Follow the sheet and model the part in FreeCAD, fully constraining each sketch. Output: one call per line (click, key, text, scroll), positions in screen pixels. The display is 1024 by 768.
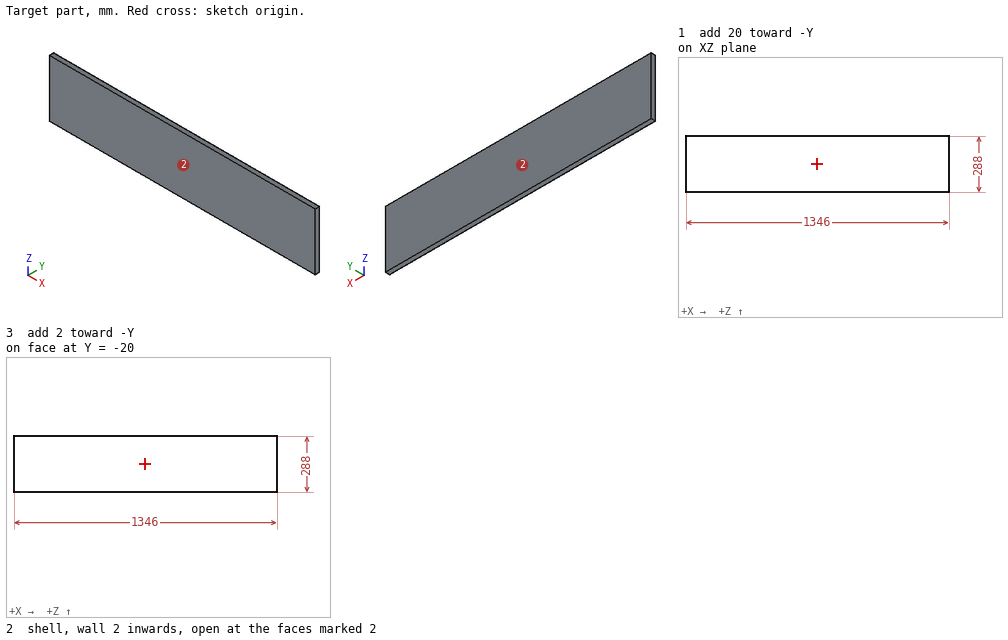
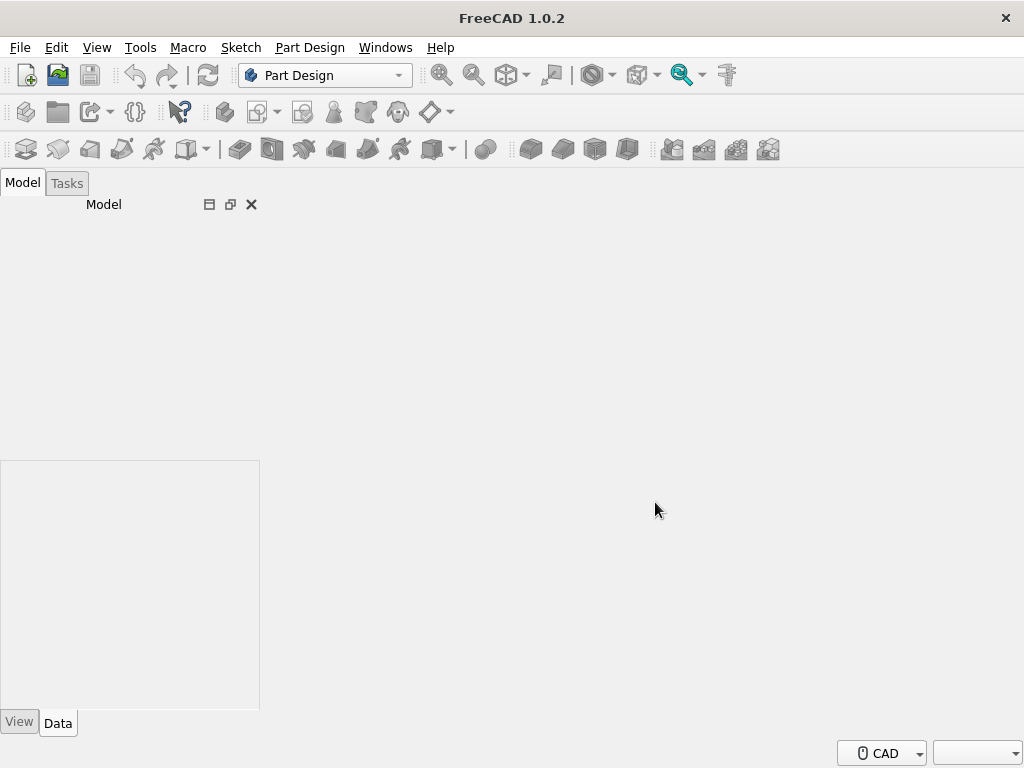
click(26, 76)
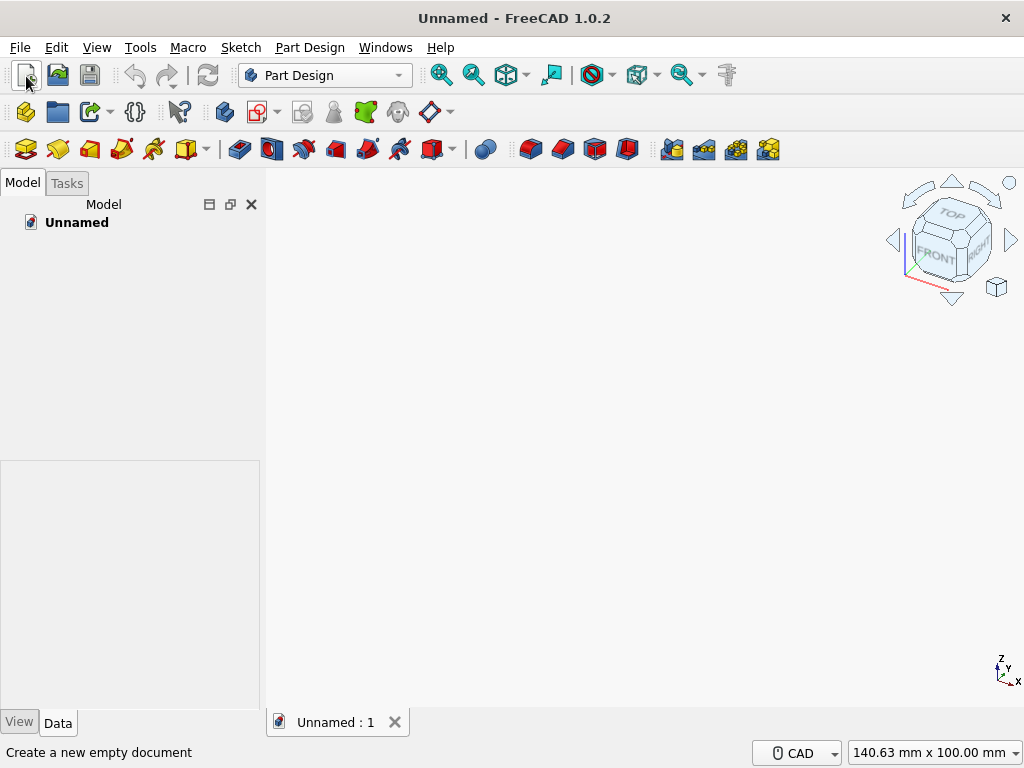
click(258, 112)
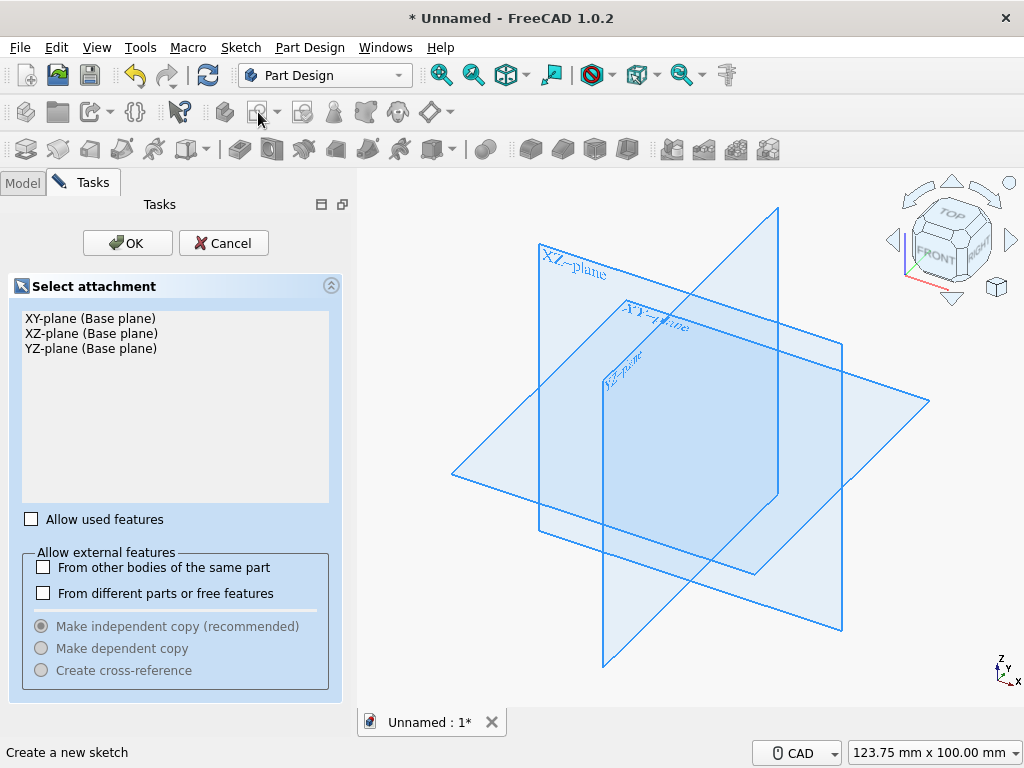
click(82, 334)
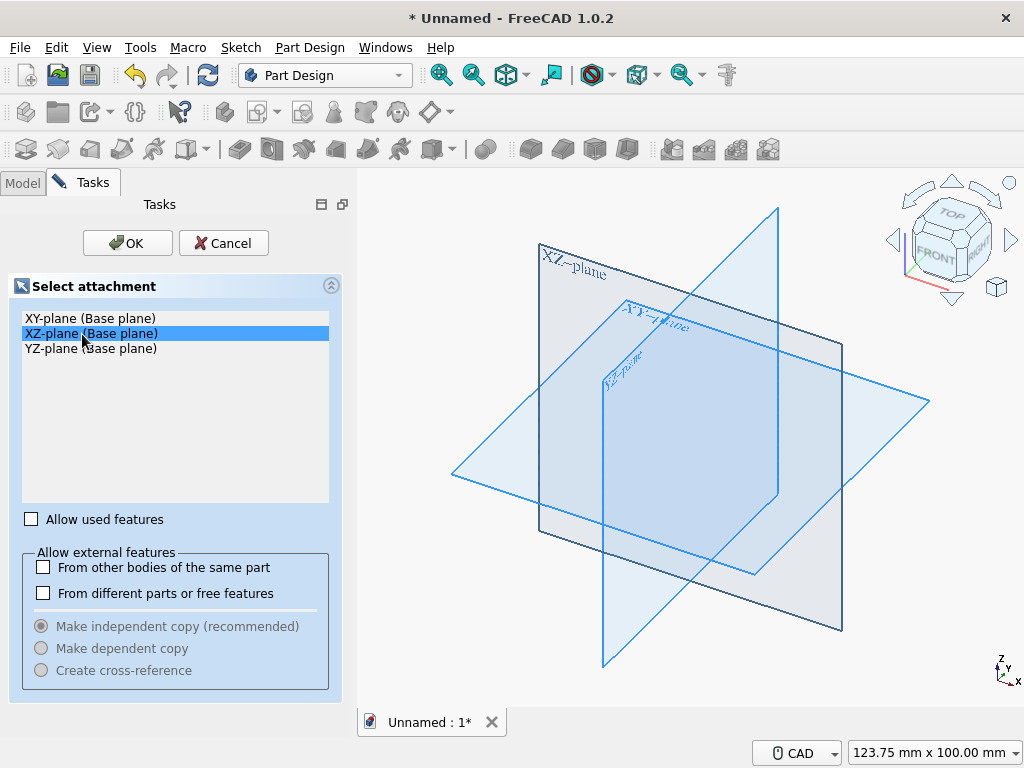
click(128, 243)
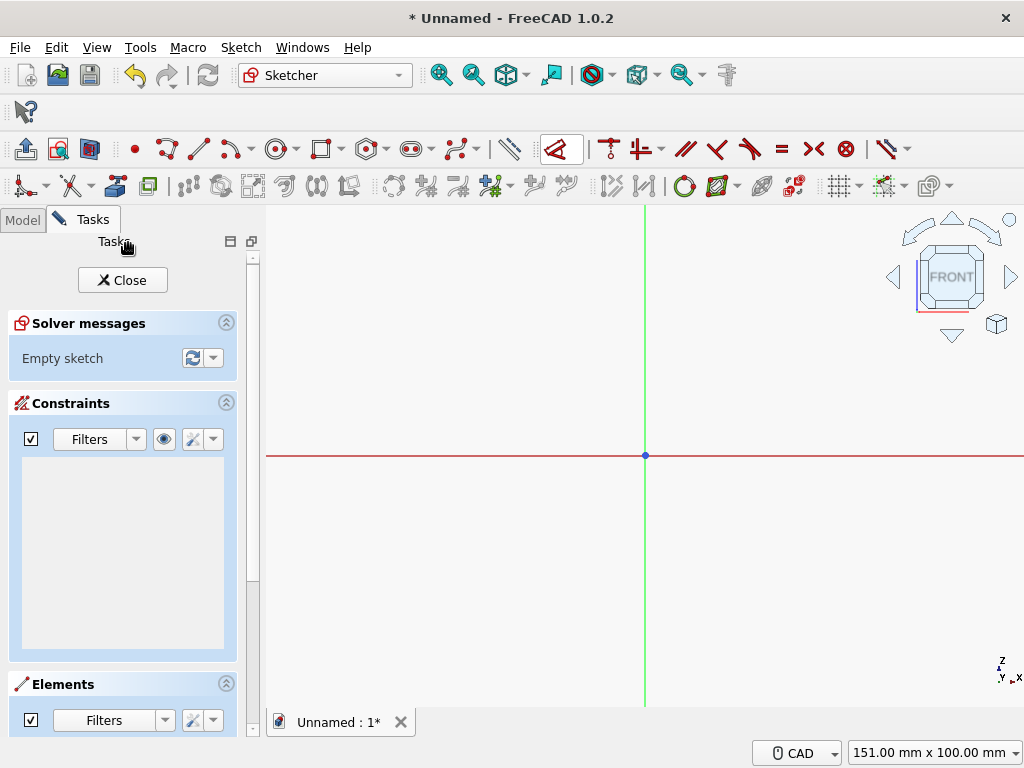
scroll(572, 456, down, 14)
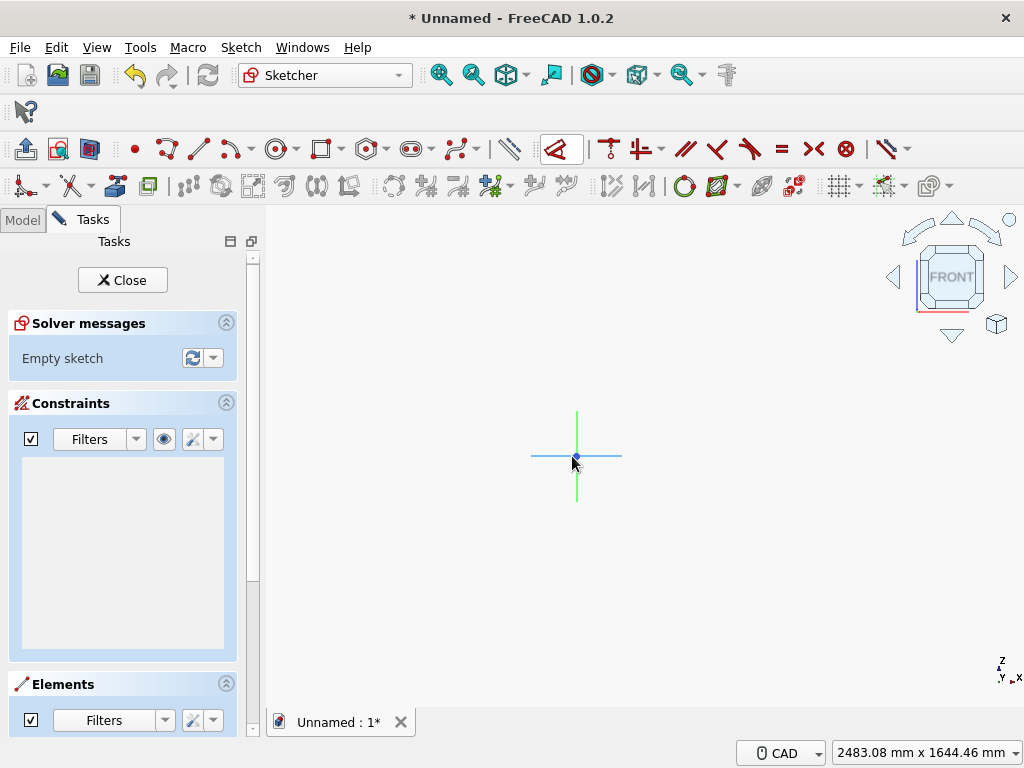
click(344, 150)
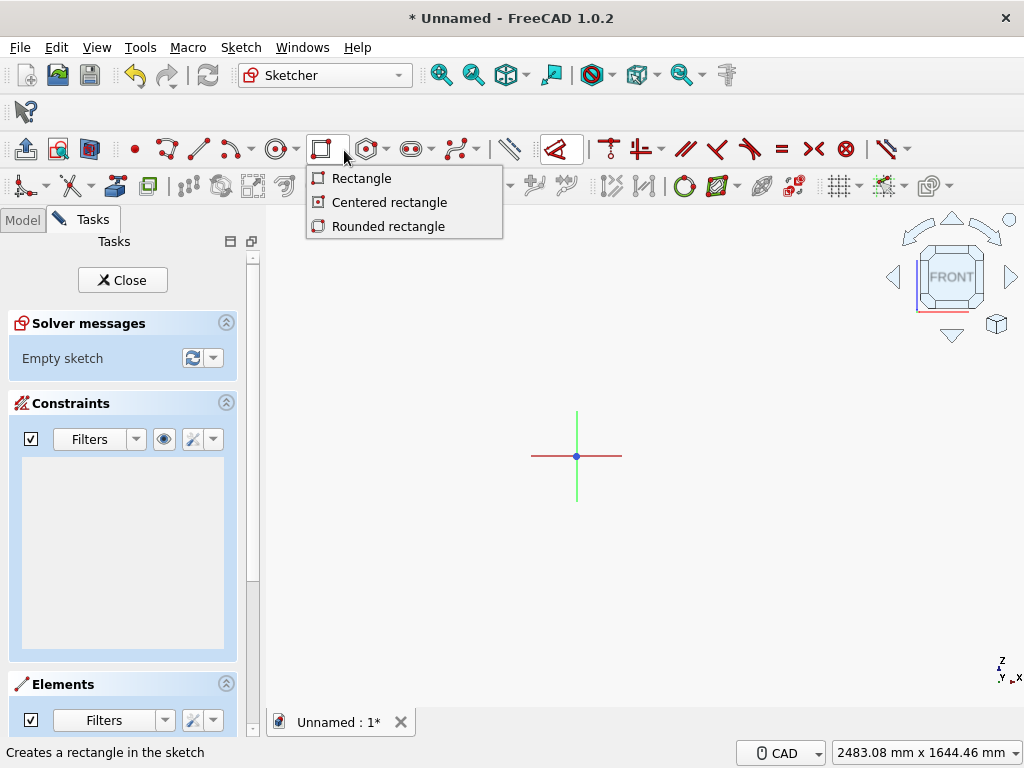
click(404, 202)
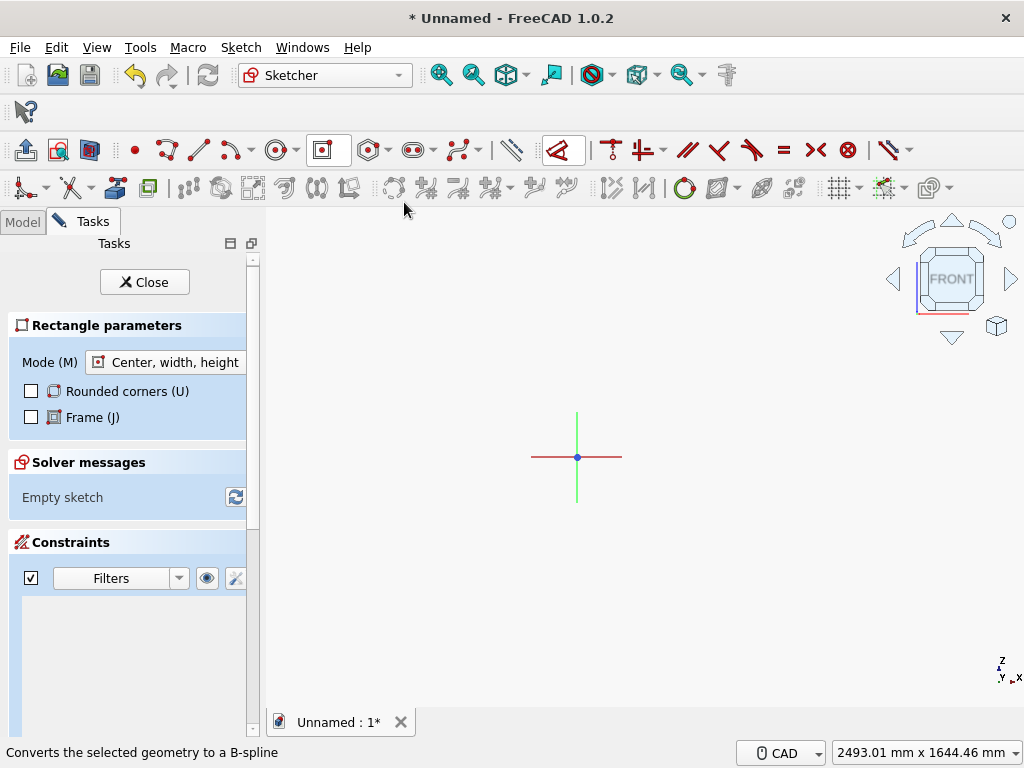
click(577, 457)
click(782, 414)
key(Escape)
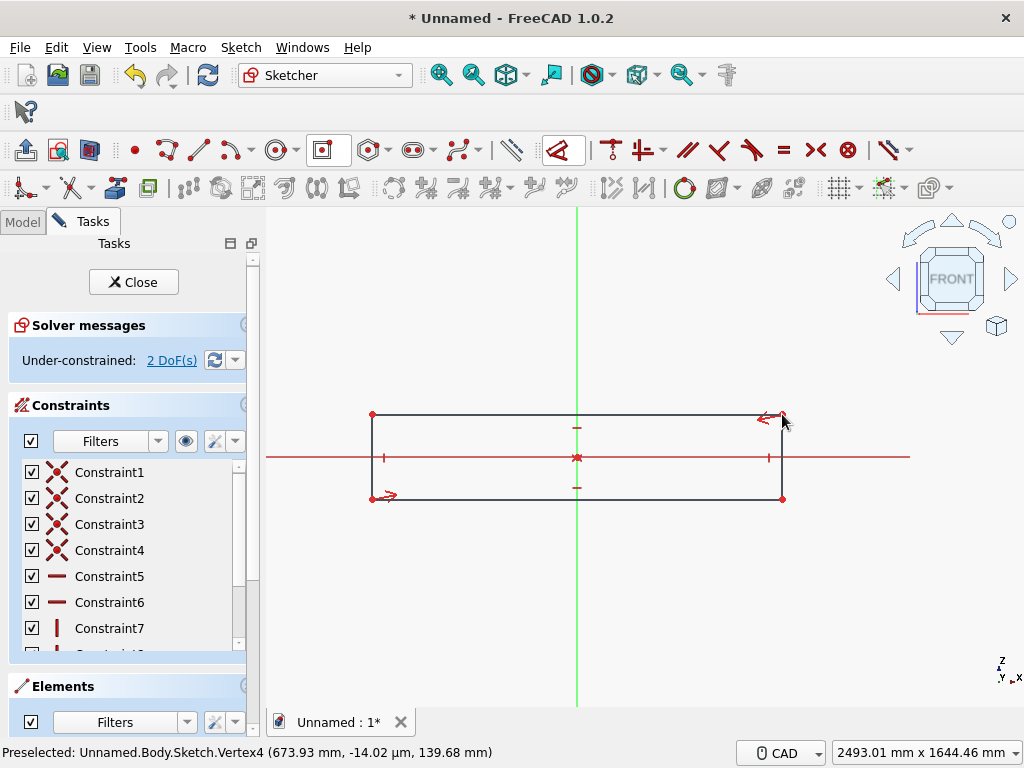
click(558, 150)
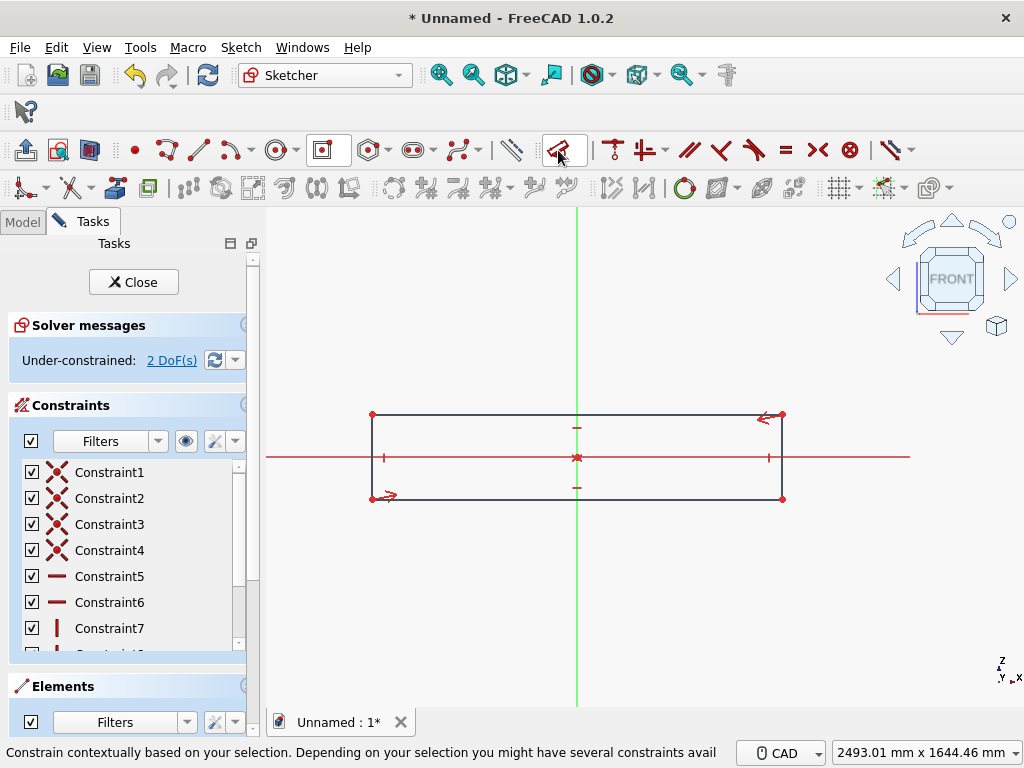
click(782, 474)
click(816, 438)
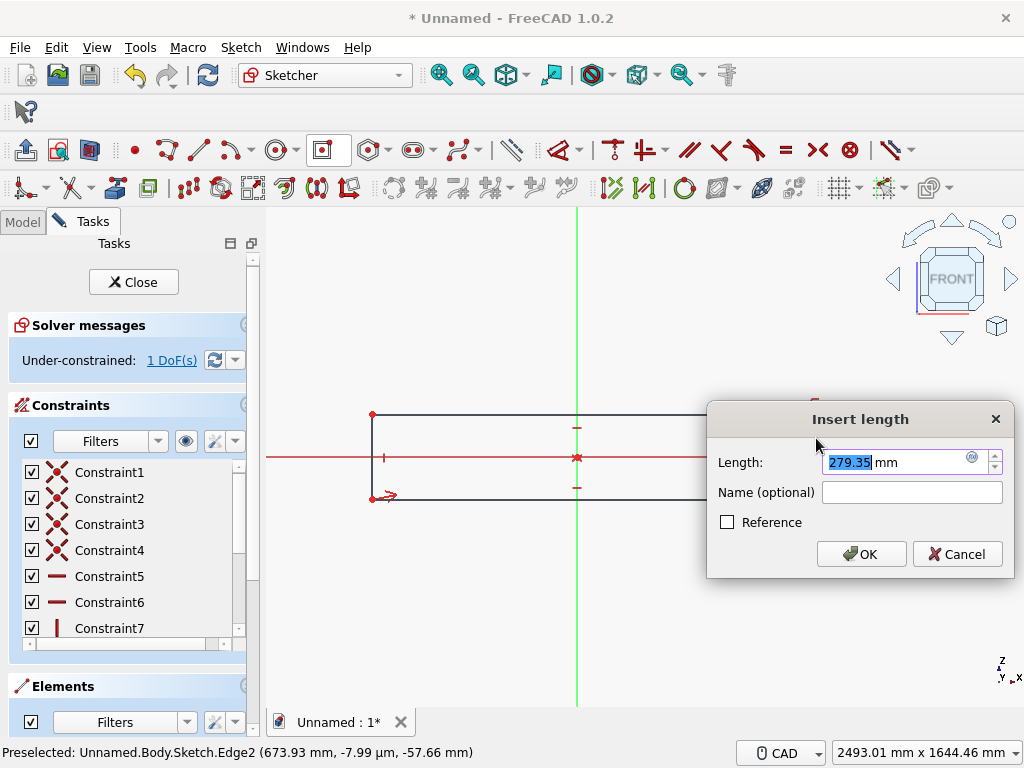
text(288)
key(Return)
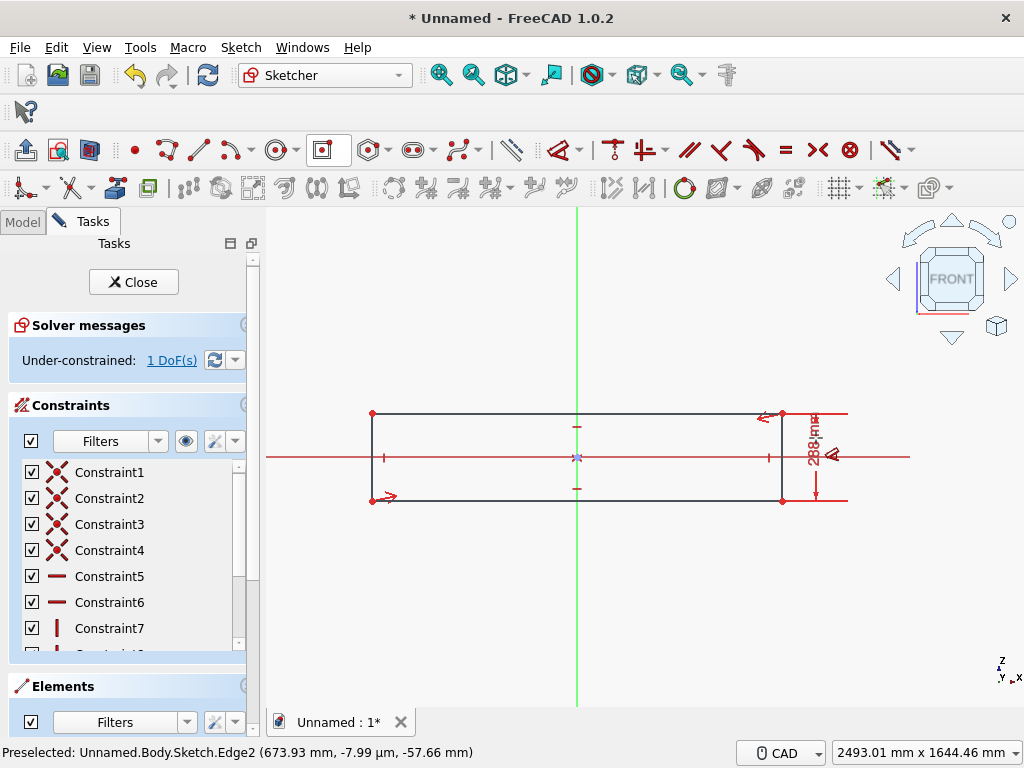
click(495, 501)
click(483, 535)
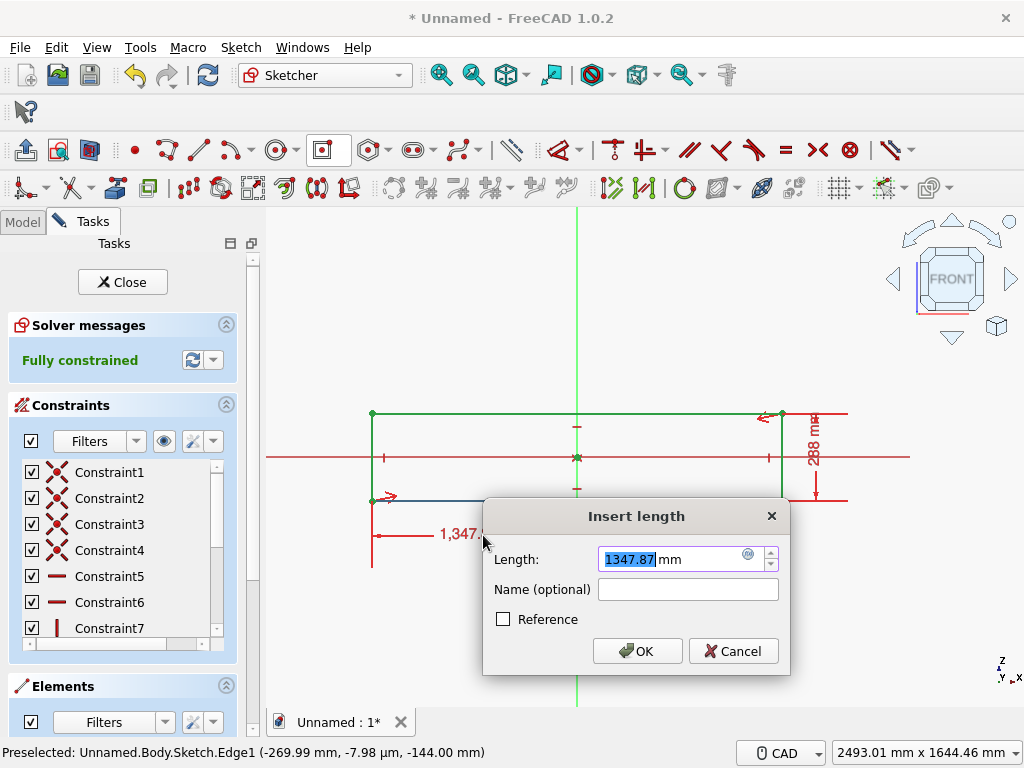
text(1346)
key(Return)
key(Escape)